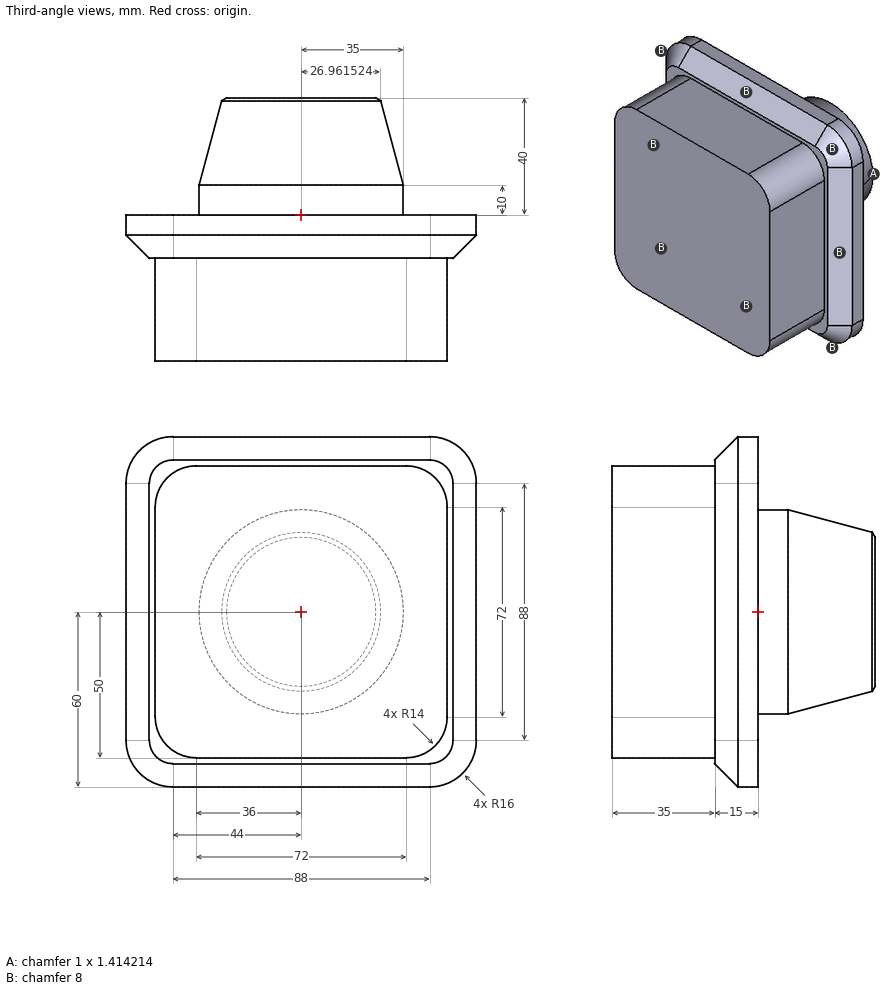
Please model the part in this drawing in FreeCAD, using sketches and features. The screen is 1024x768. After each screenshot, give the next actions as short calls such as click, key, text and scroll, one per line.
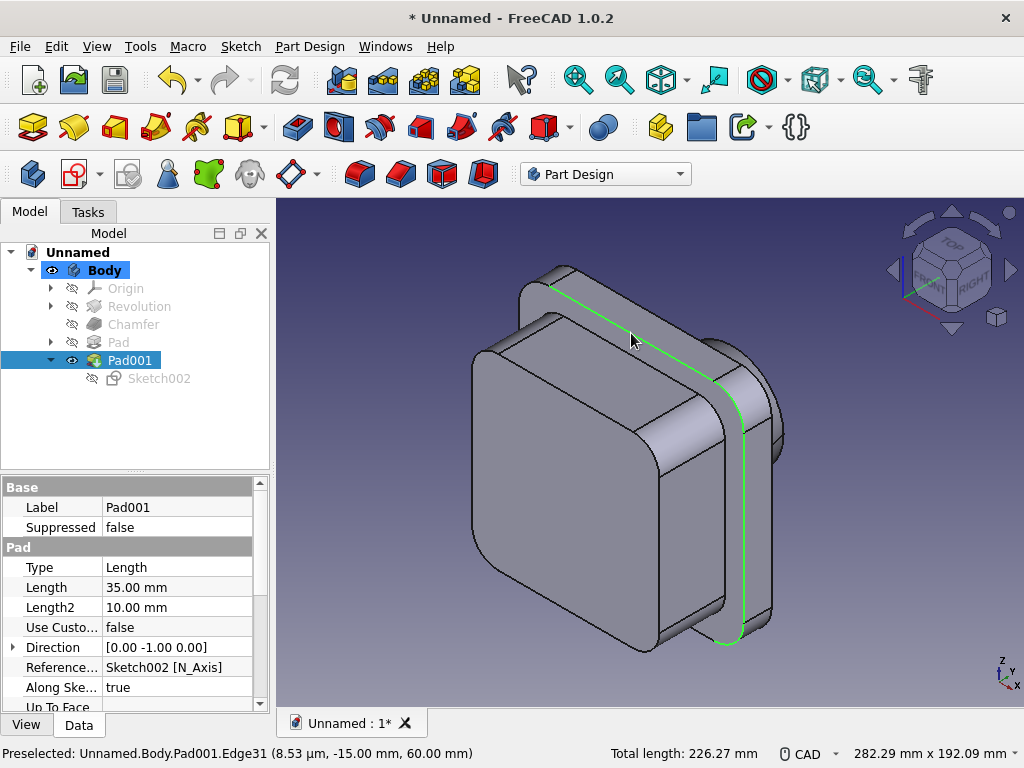
click(531, 281, ctrl)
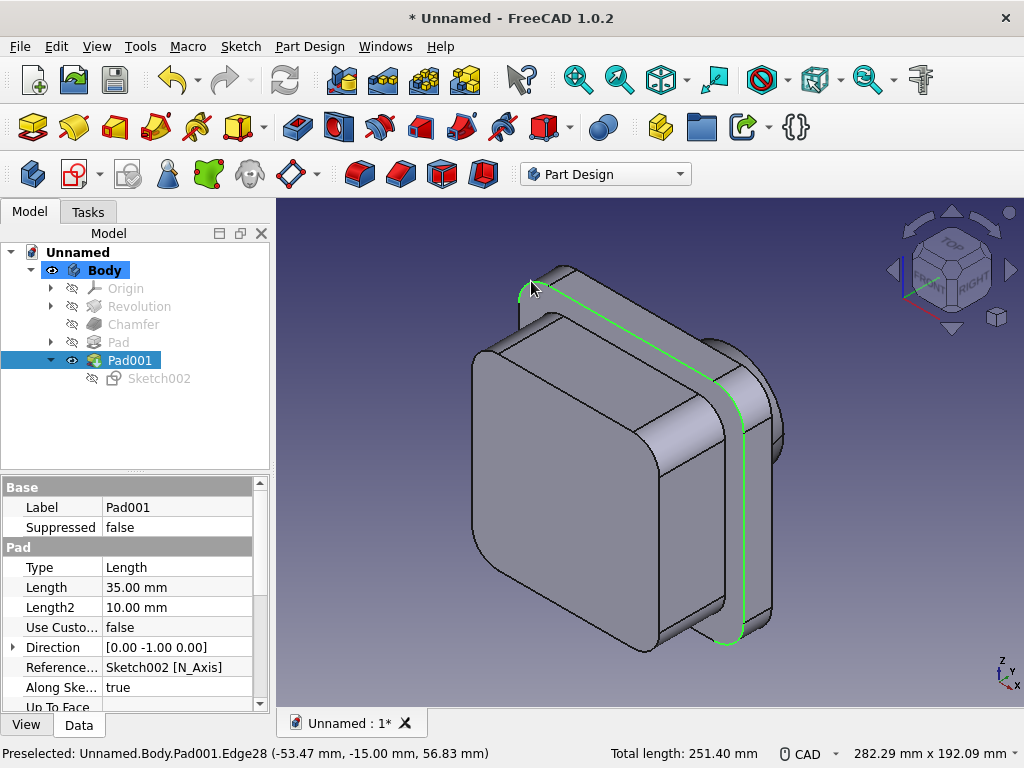
key(2)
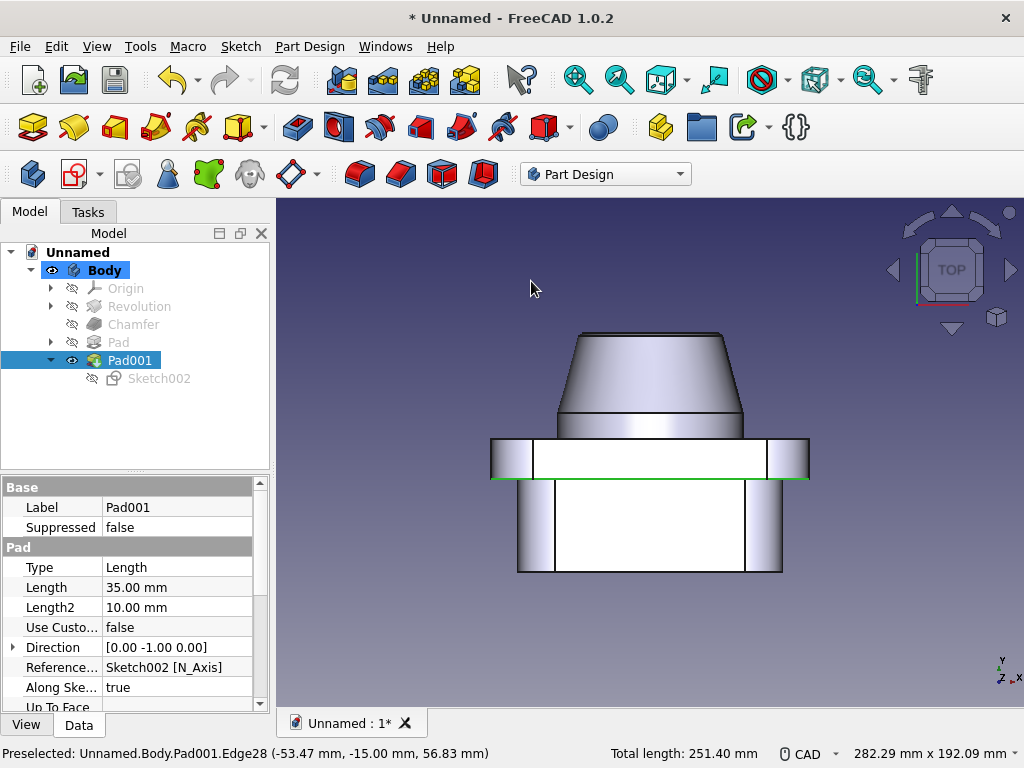
key(0)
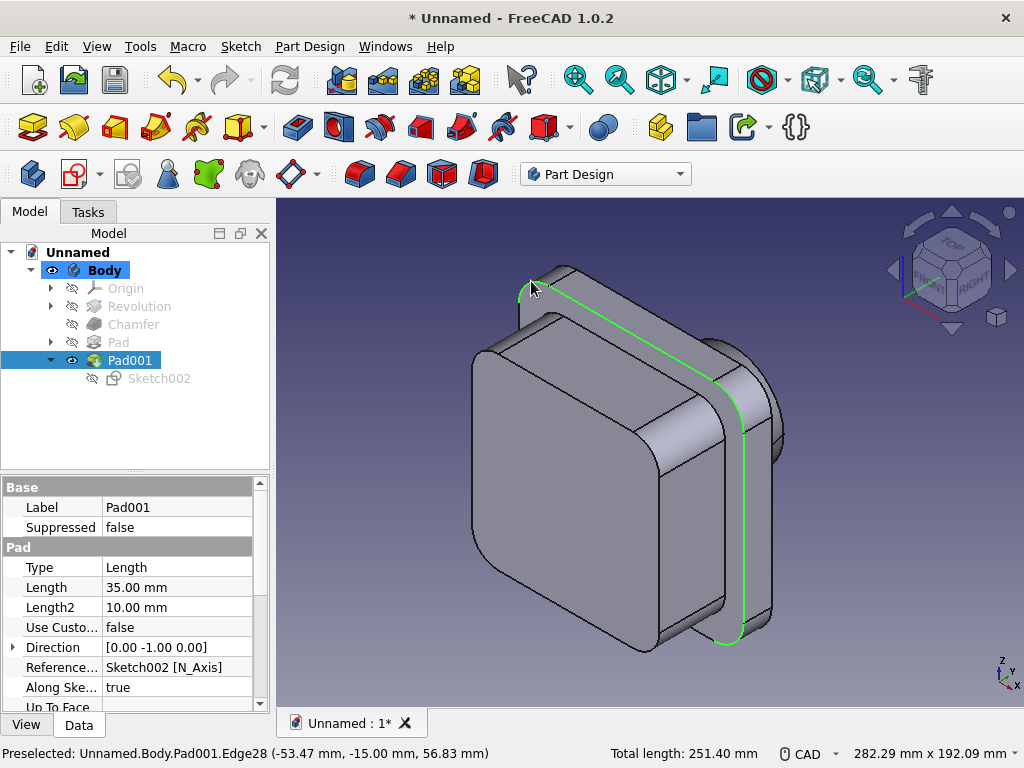
key(1)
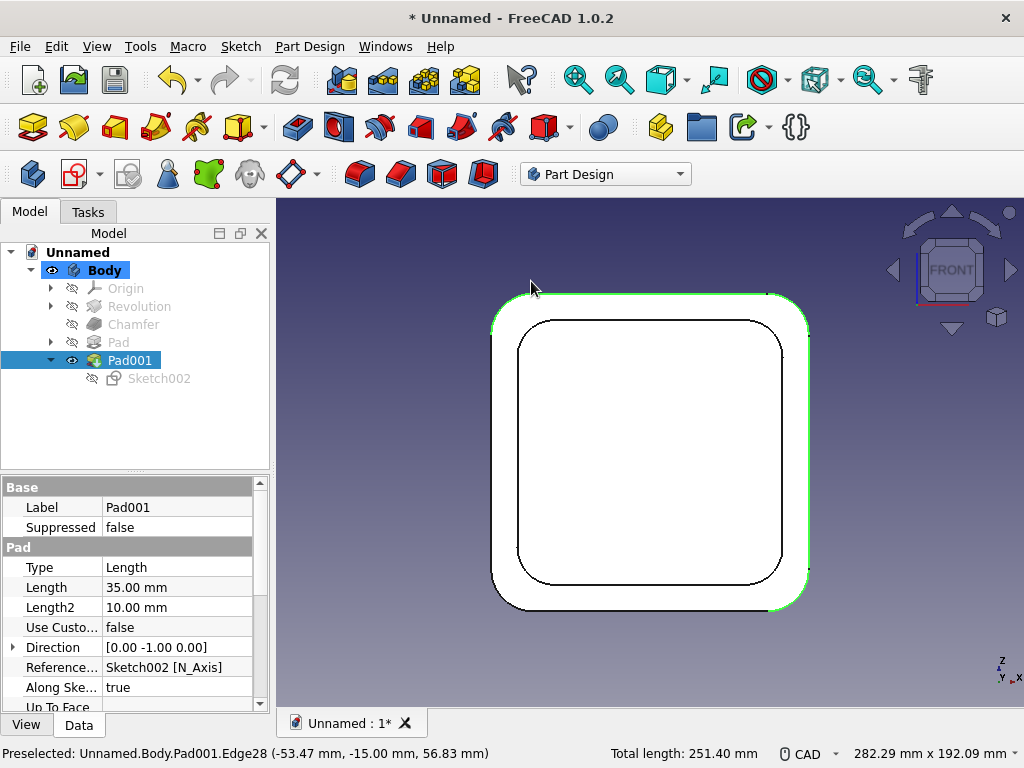
click(503, 598, ctrl)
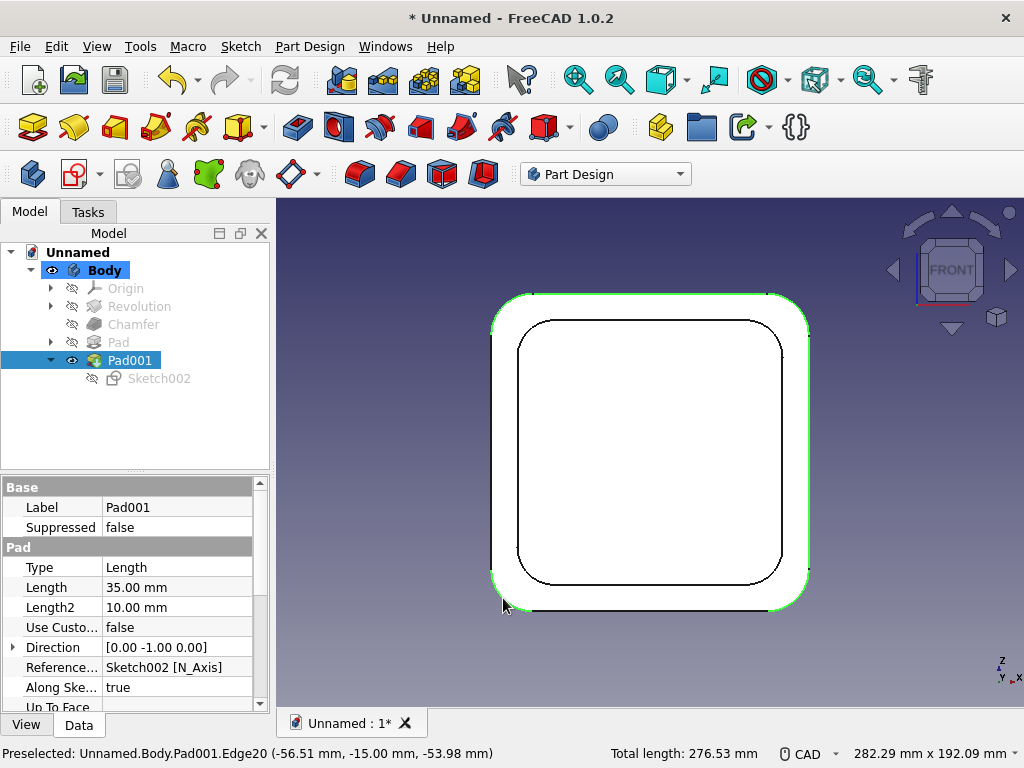
click(650, 610, ctrl)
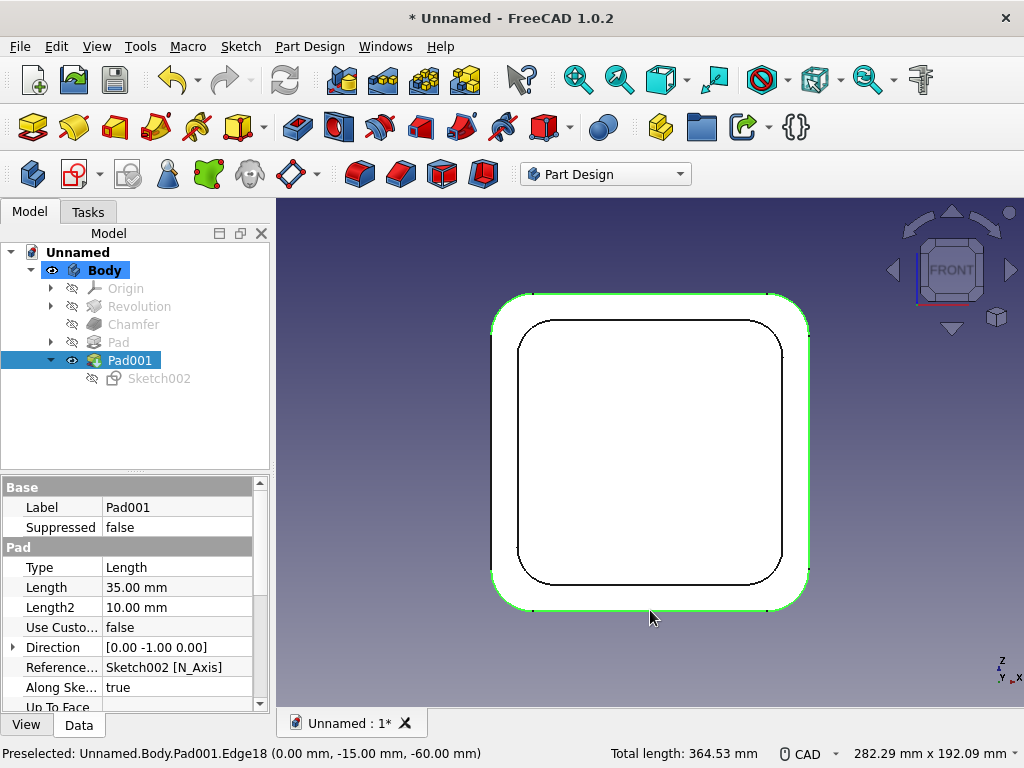
click(491, 451, ctrl)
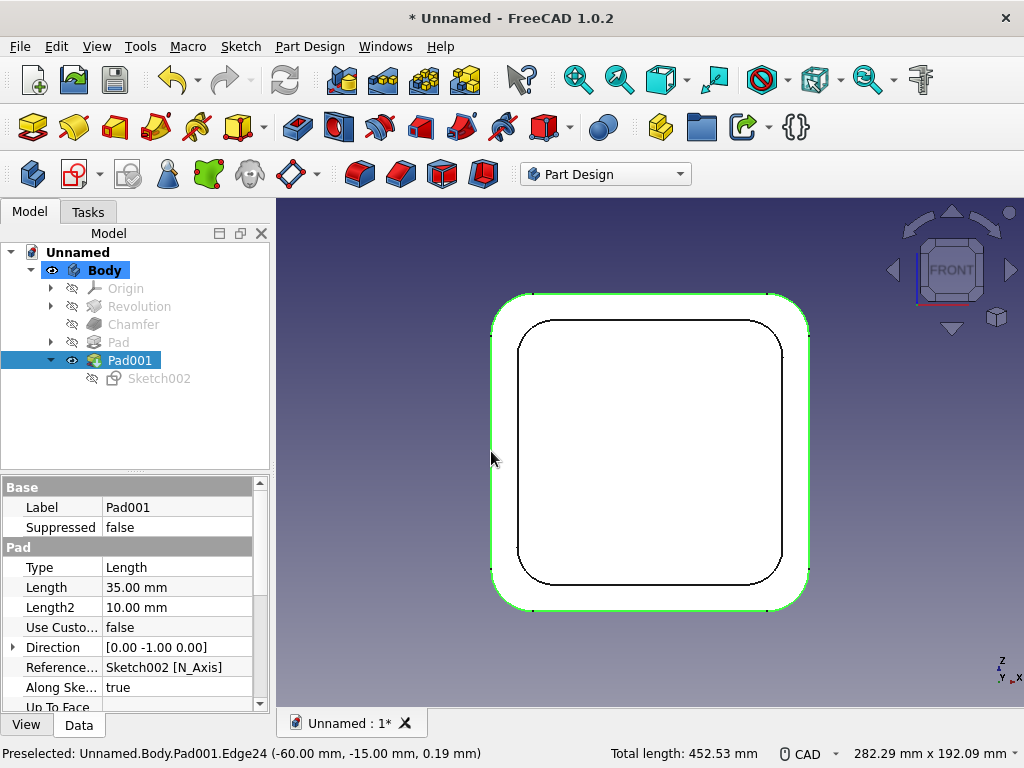
click(401, 174)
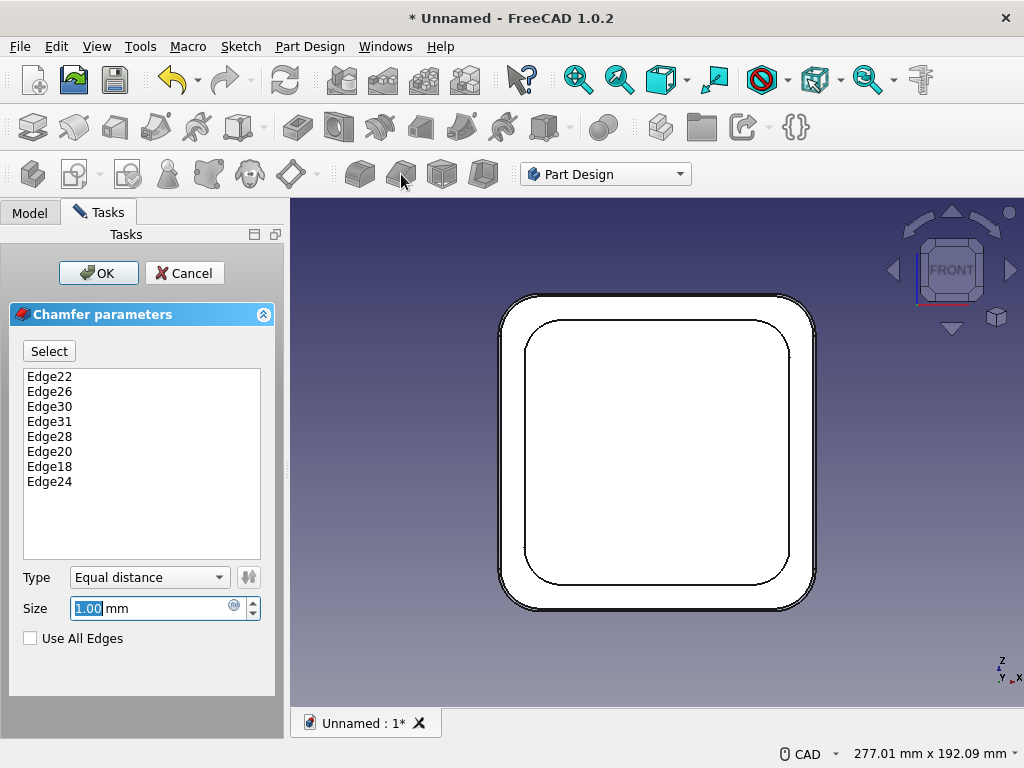
text(8)
key(Tab)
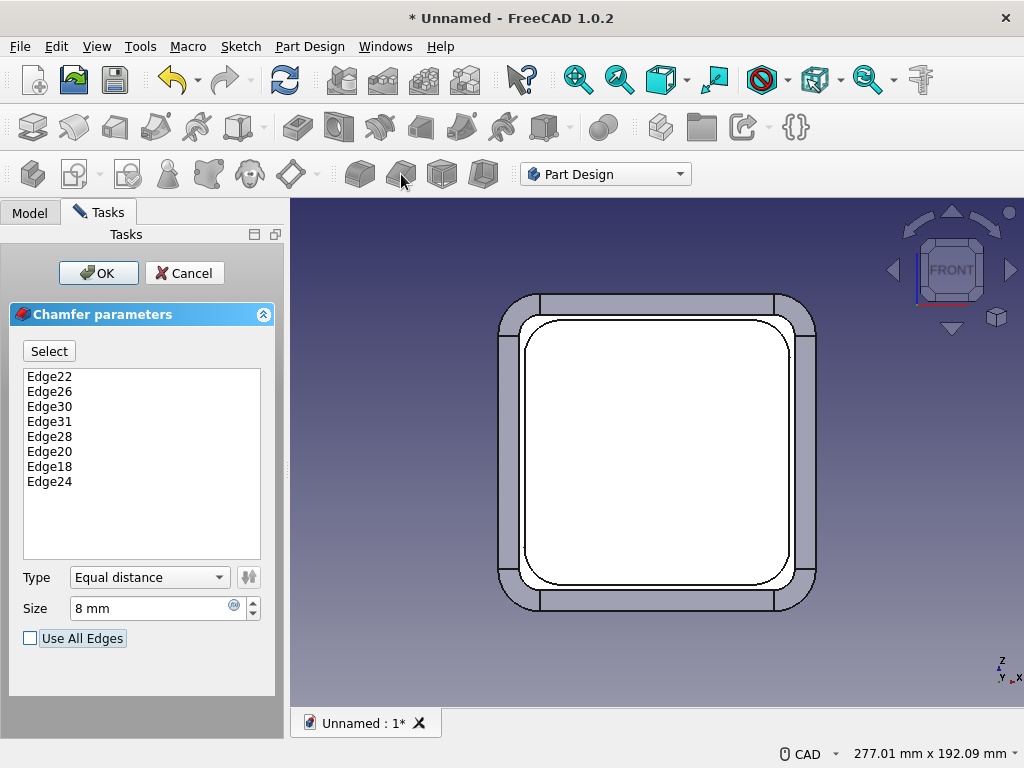
click(99, 273)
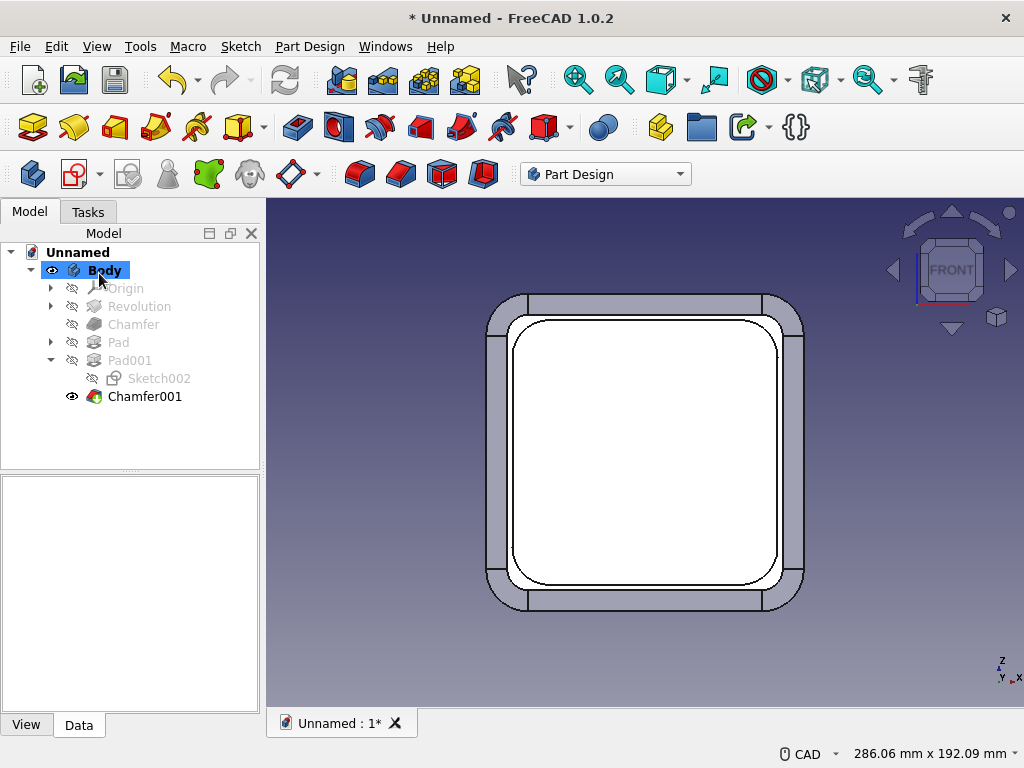
key(0)